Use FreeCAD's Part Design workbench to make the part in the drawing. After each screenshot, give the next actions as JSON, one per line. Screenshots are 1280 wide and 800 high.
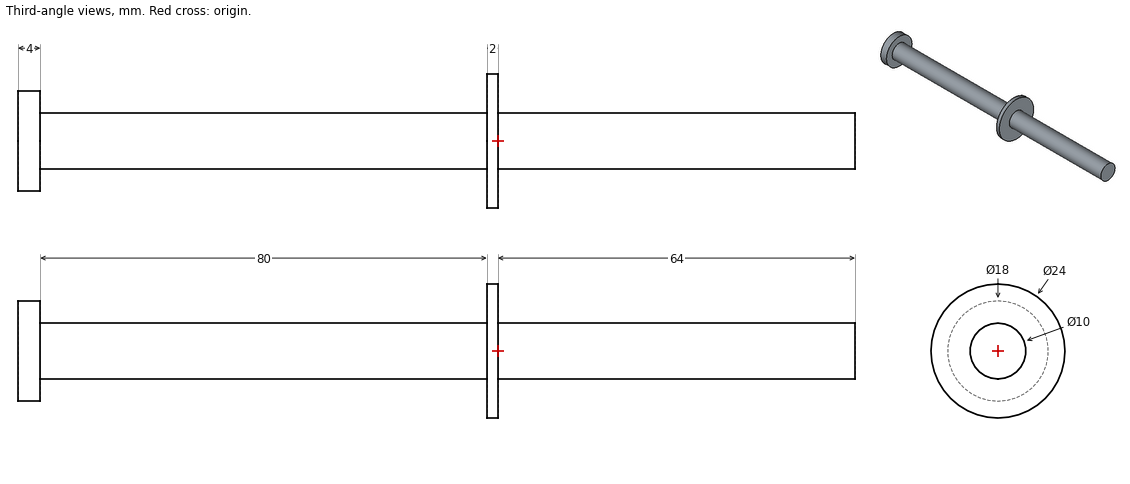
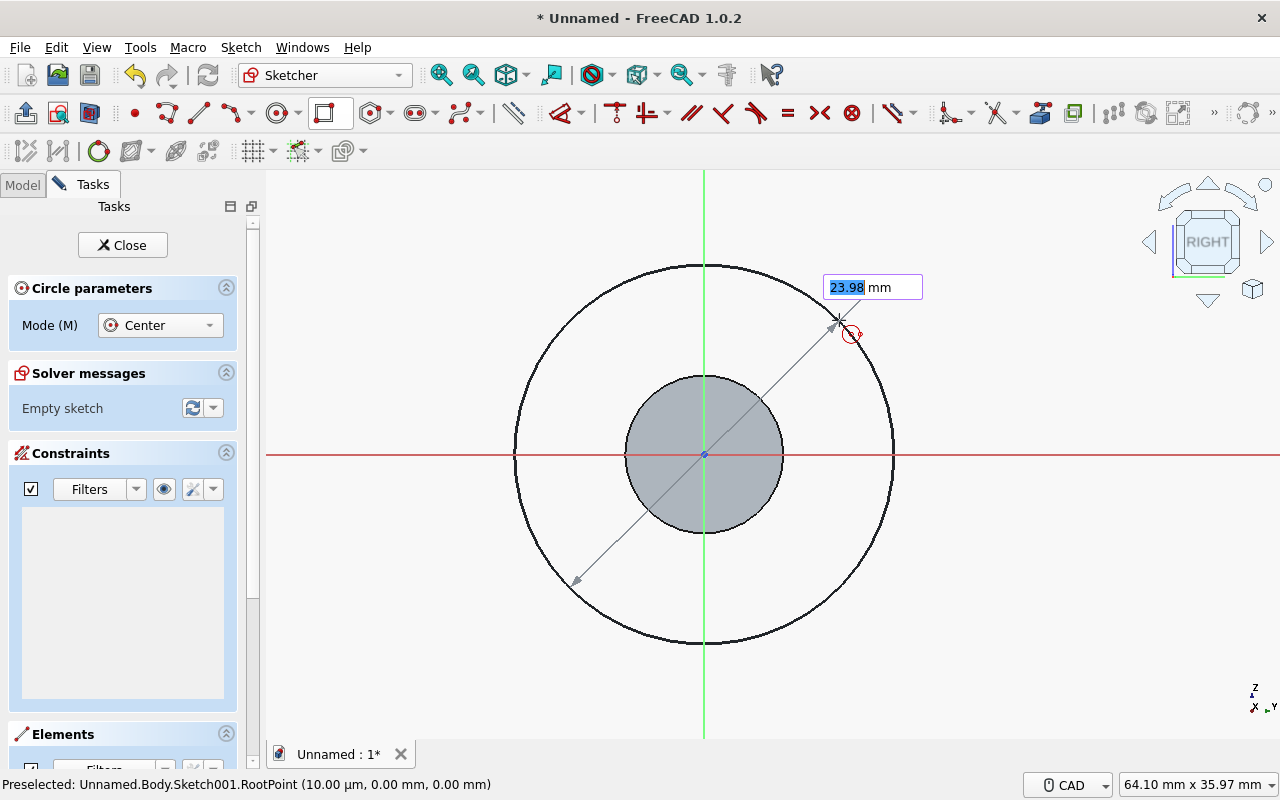
{"action": "type", "text": "24"}
{"action": "key", "text": "Return"}
{"action": "key", "text": "Escape"}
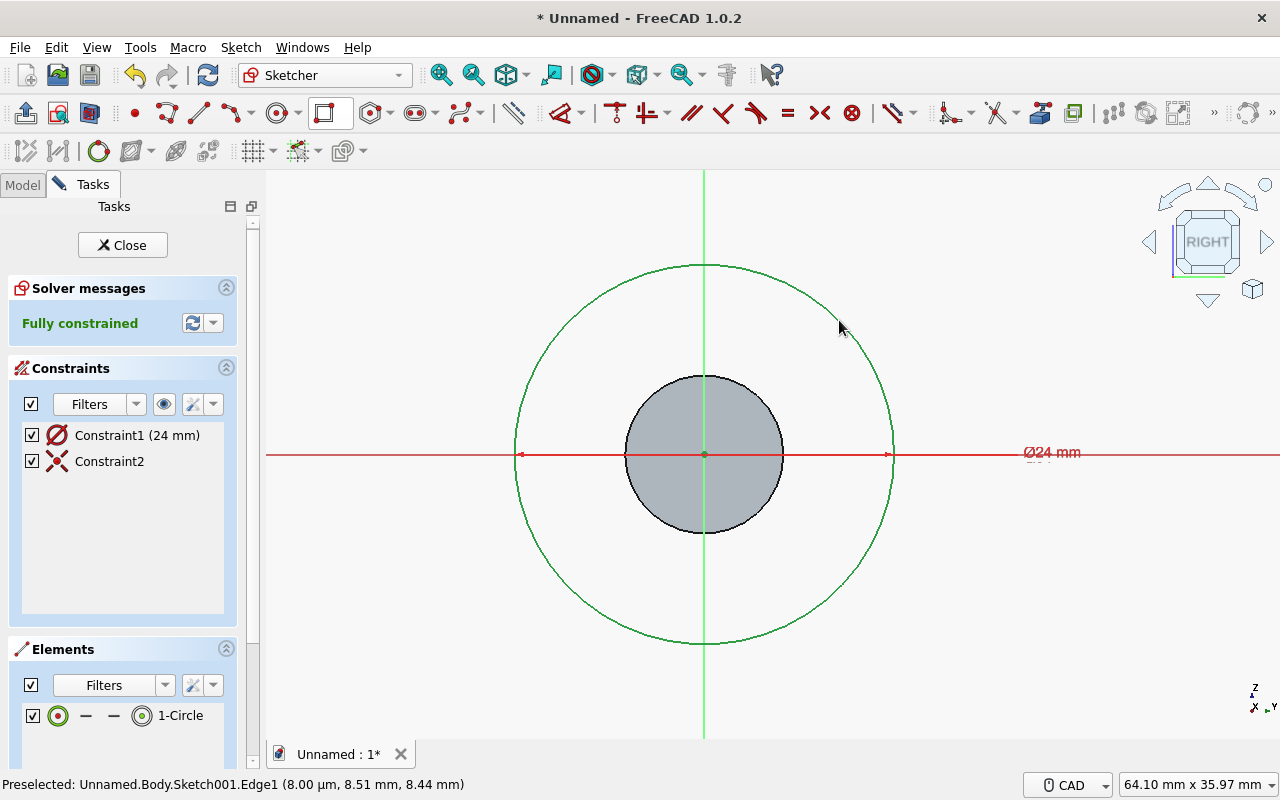
{"action": "left_click", "coordinate": [123, 245]}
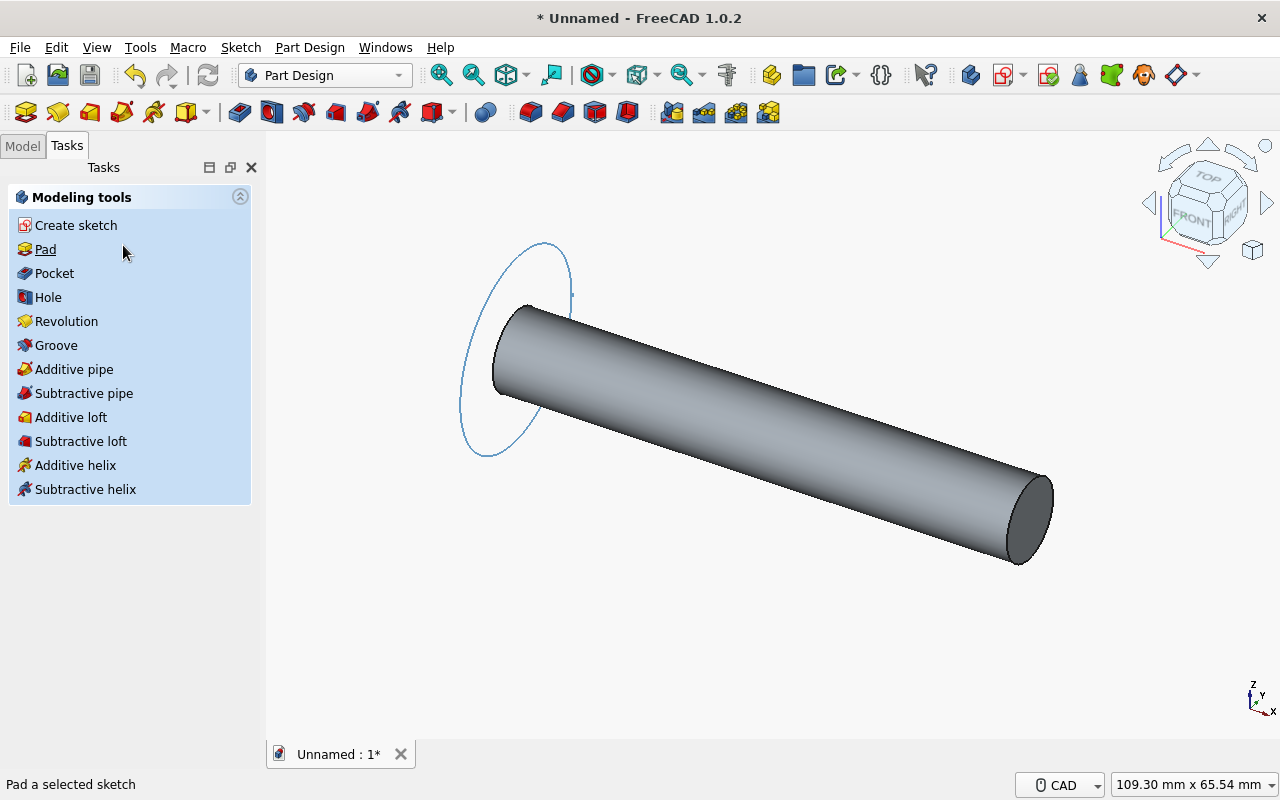
{"action": "left_click", "coordinate": [26, 112]}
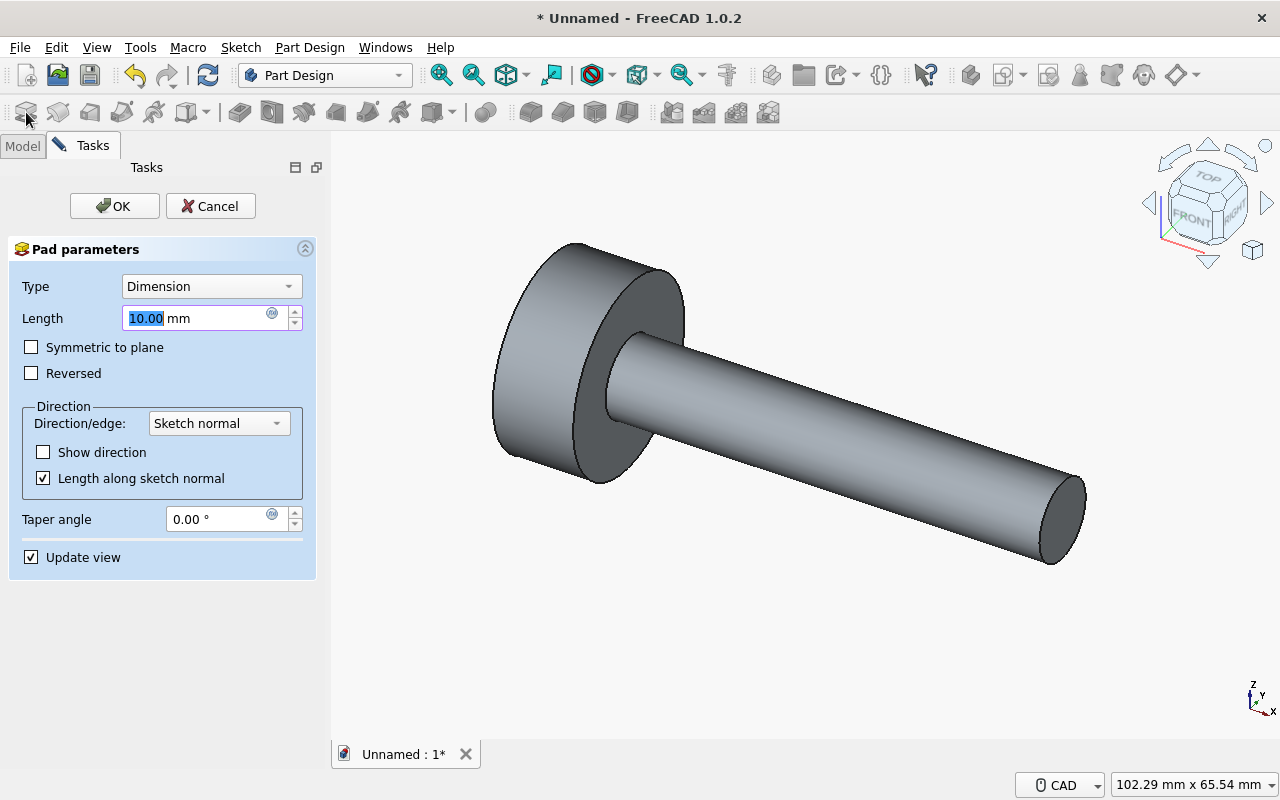
{"action": "type", "text": "2"}
{"action": "key", "text": "Tab"}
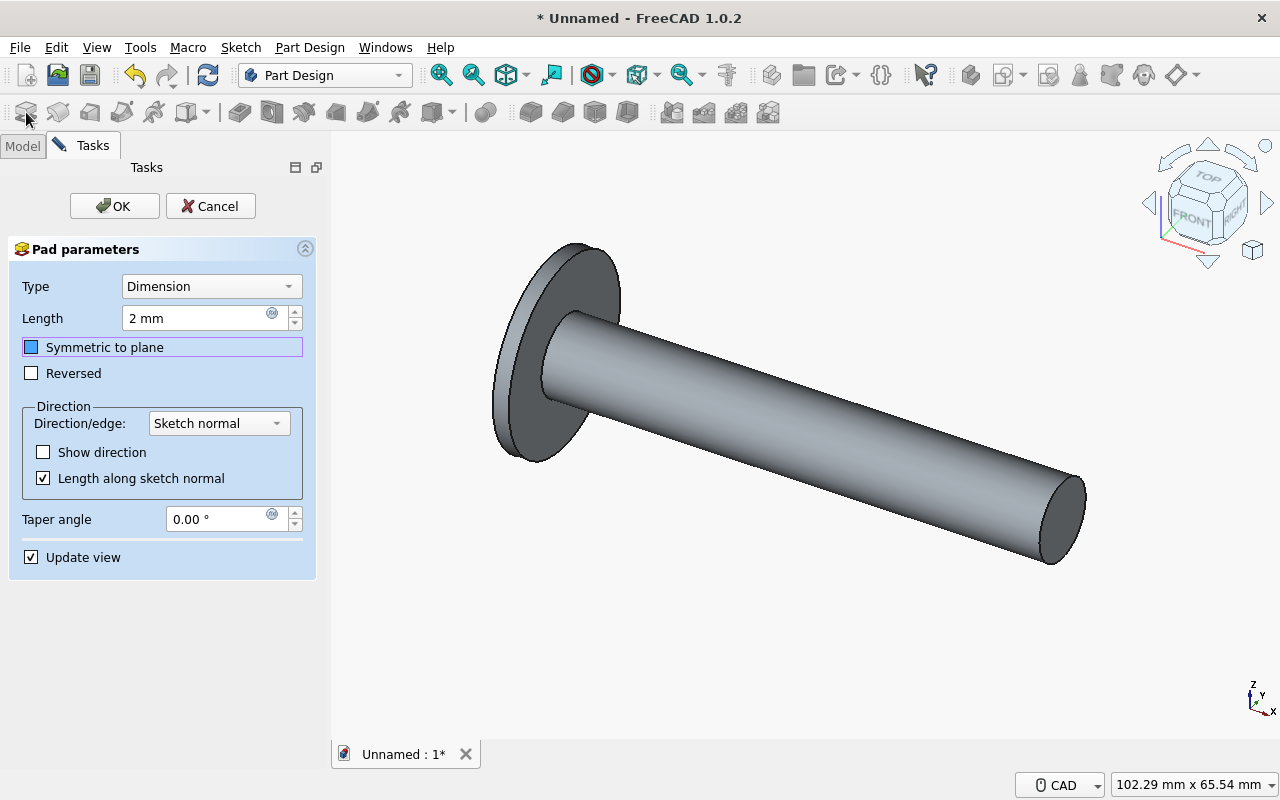
{"action": "left_click", "coordinate": [30, 373]}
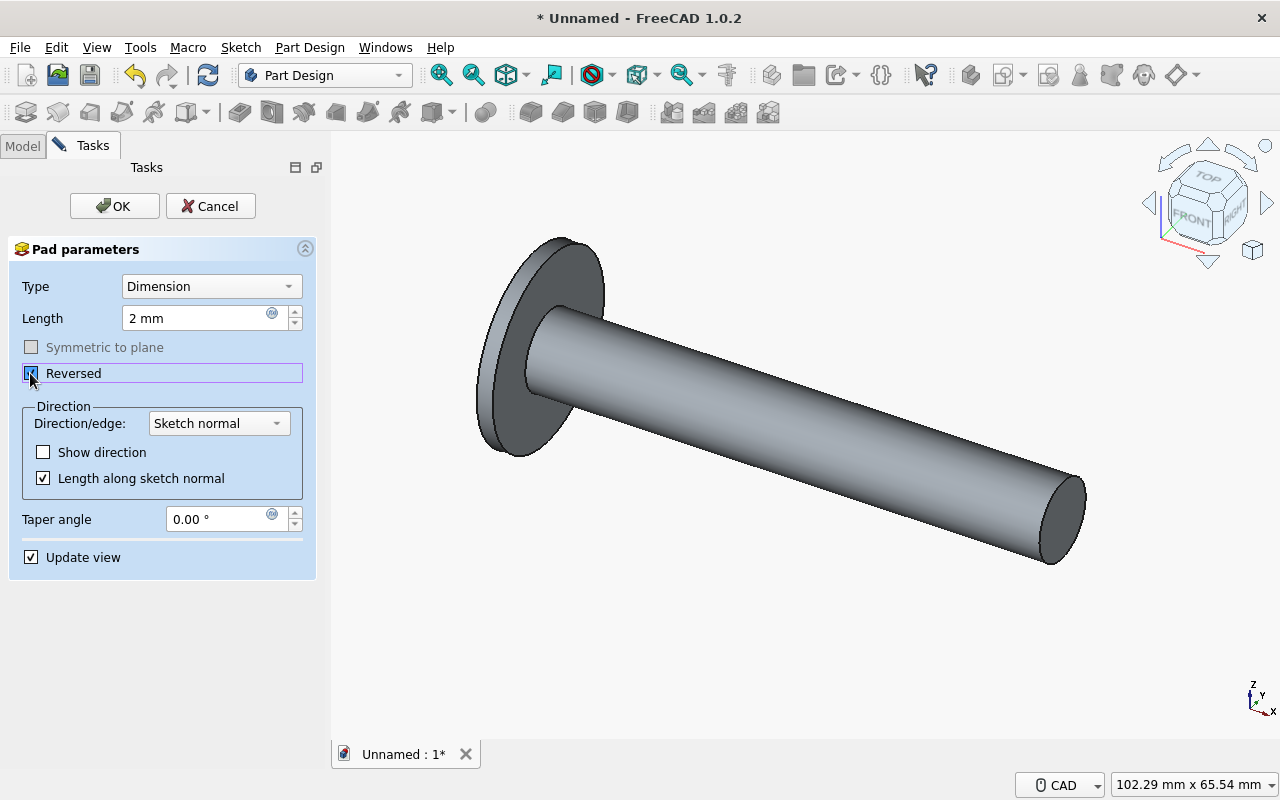
{"action": "left_click", "coordinate": [115, 206]}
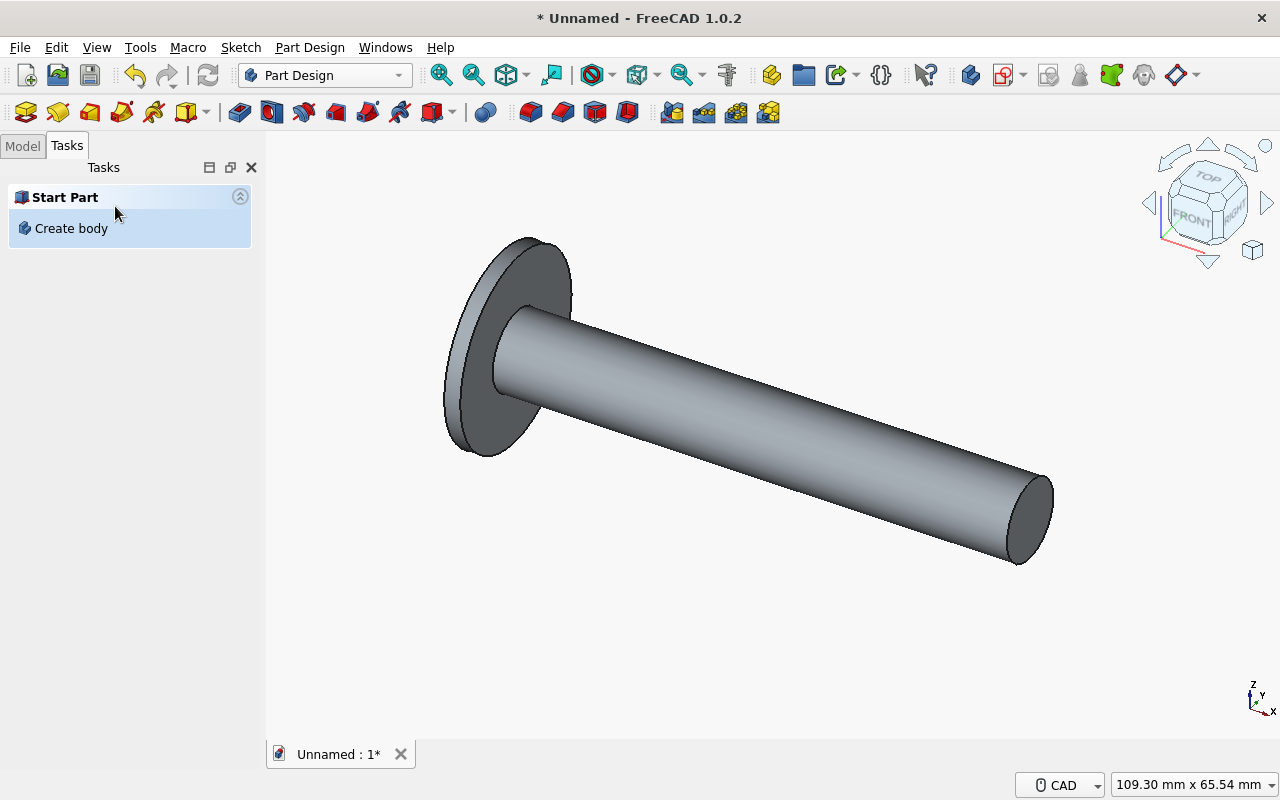
{"action": "left_click", "coordinate": [23, 145]}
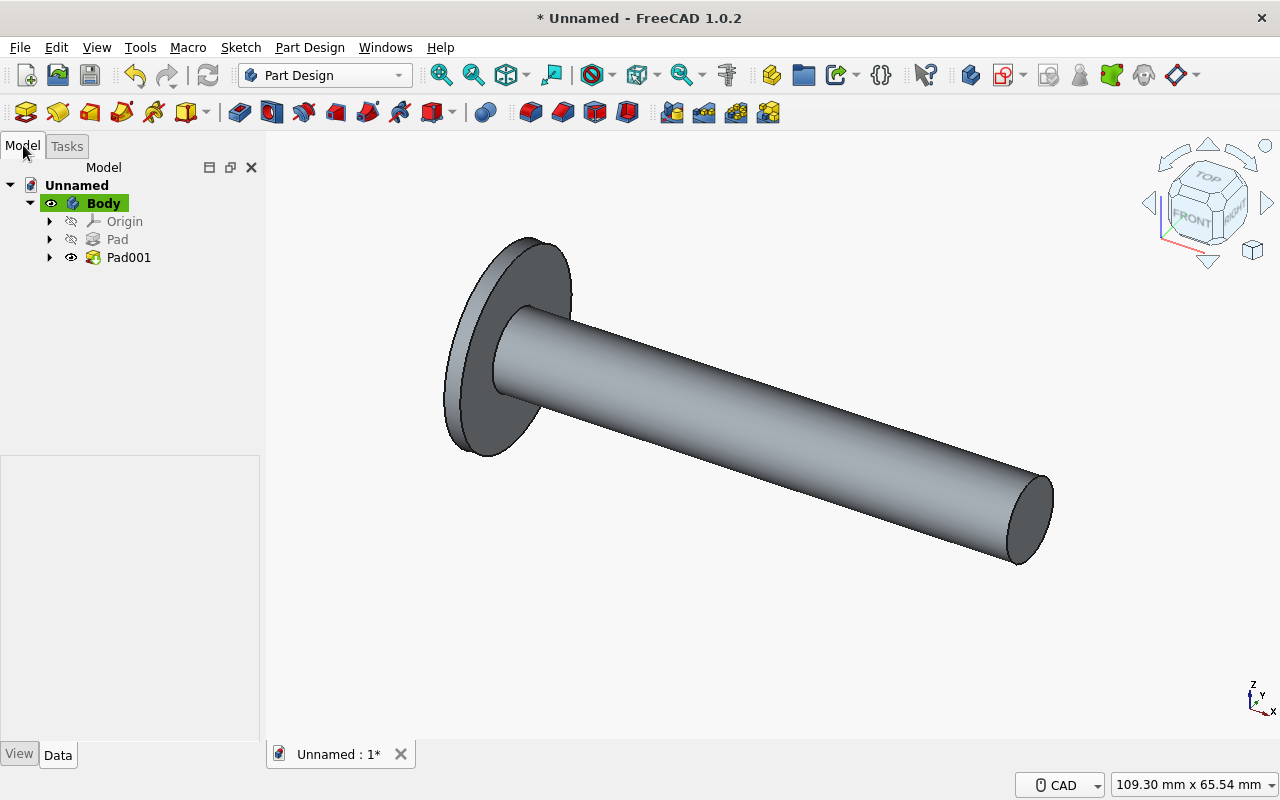
{"action": "left_click", "coordinate": [50, 221]}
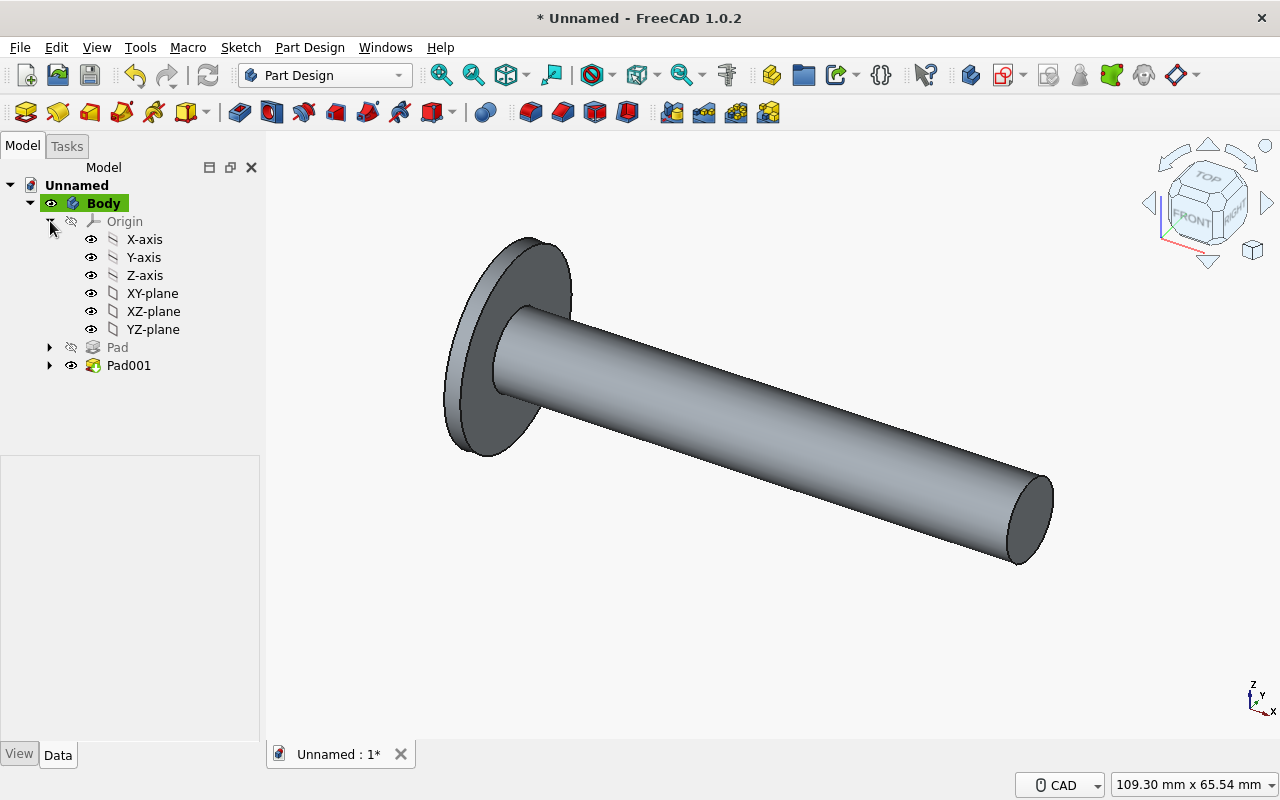
{"action": "left_click", "coordinate": [136, 329]}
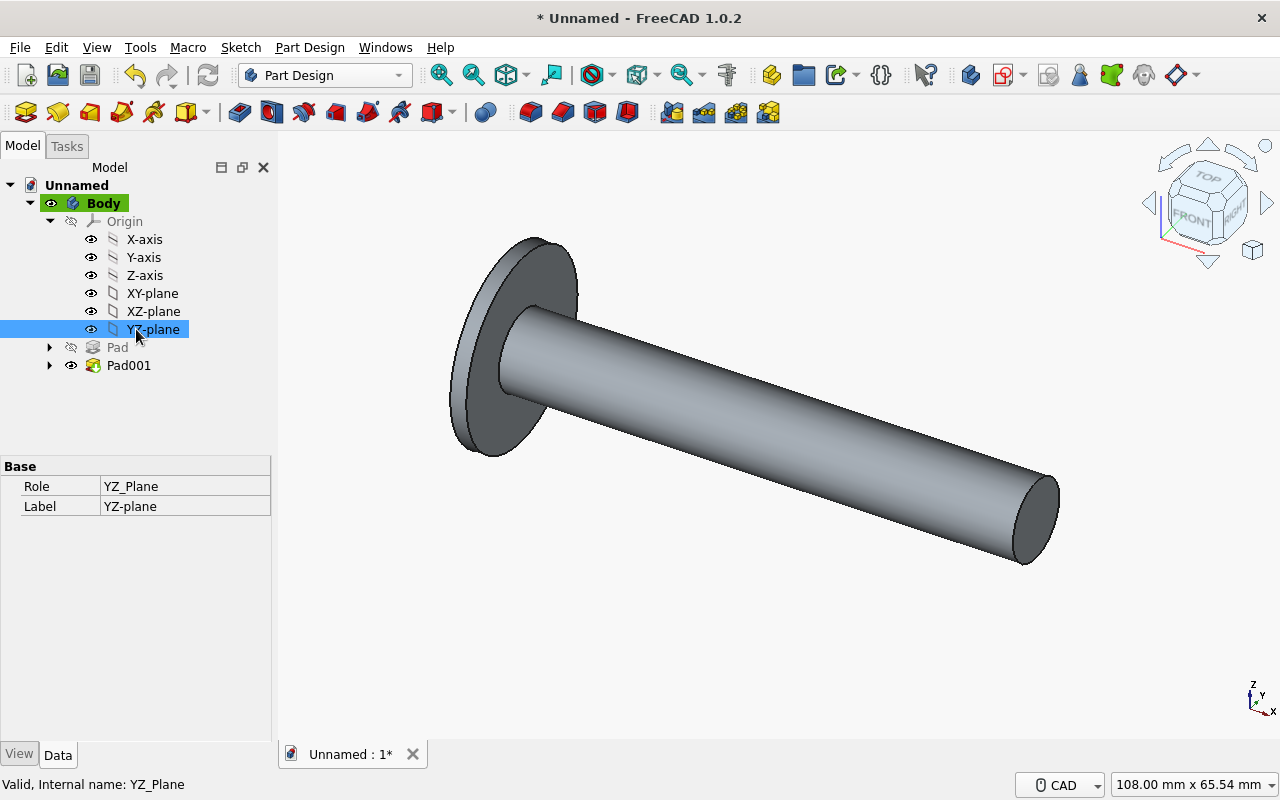
{"action": "left_click", "coordinate": [1176, 76]}